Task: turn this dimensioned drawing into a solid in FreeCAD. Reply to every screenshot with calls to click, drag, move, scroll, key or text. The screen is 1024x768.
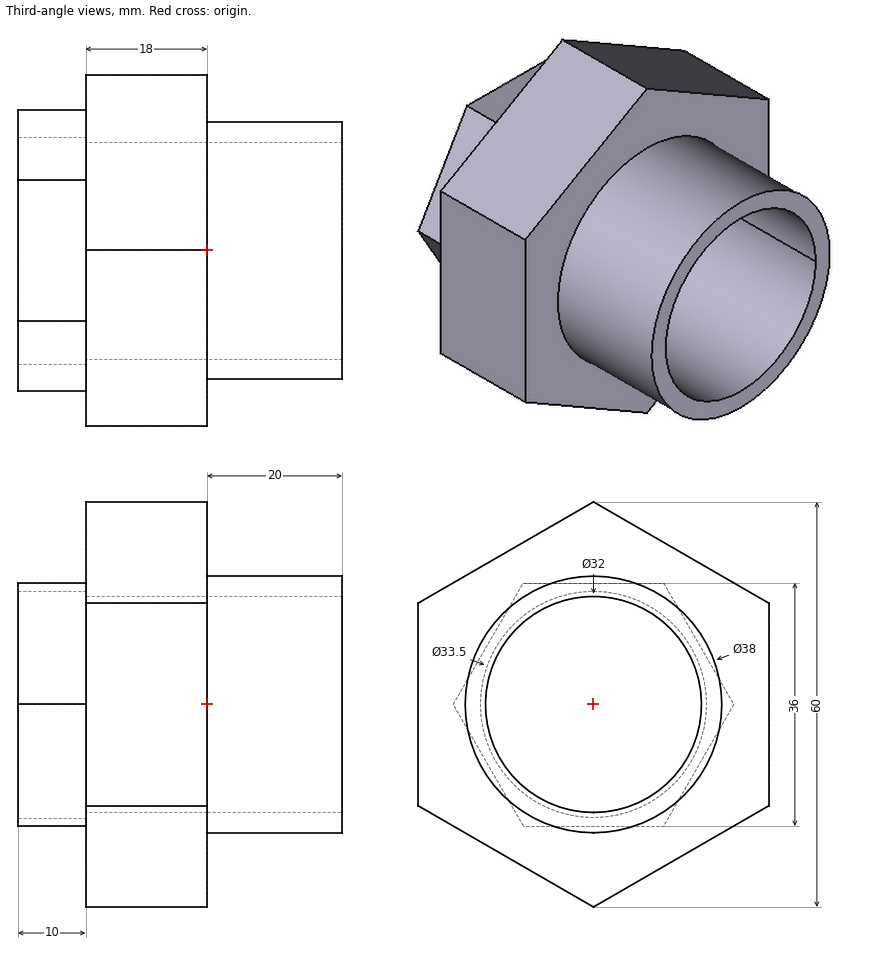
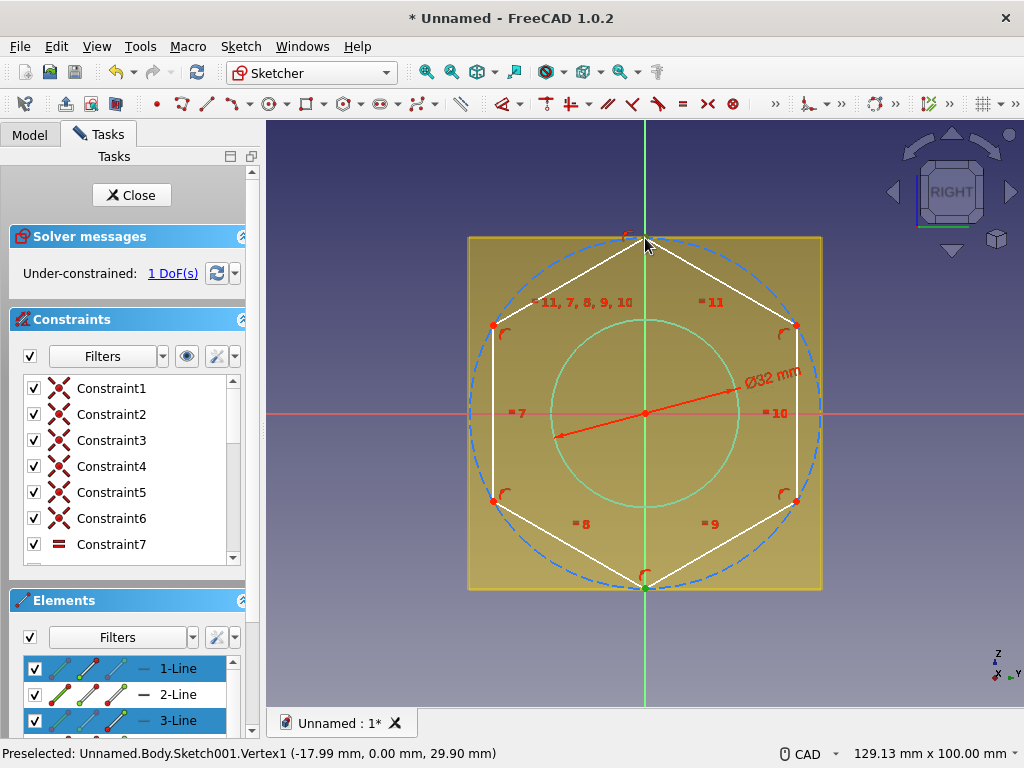
key(i)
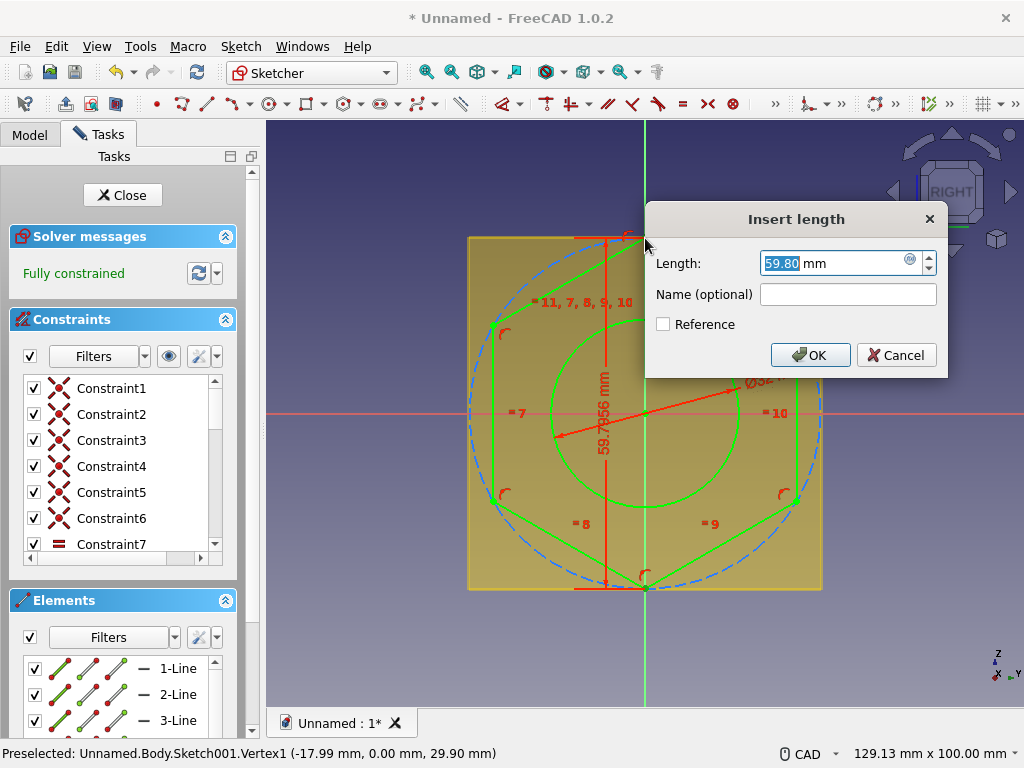
text(60)
key(Return)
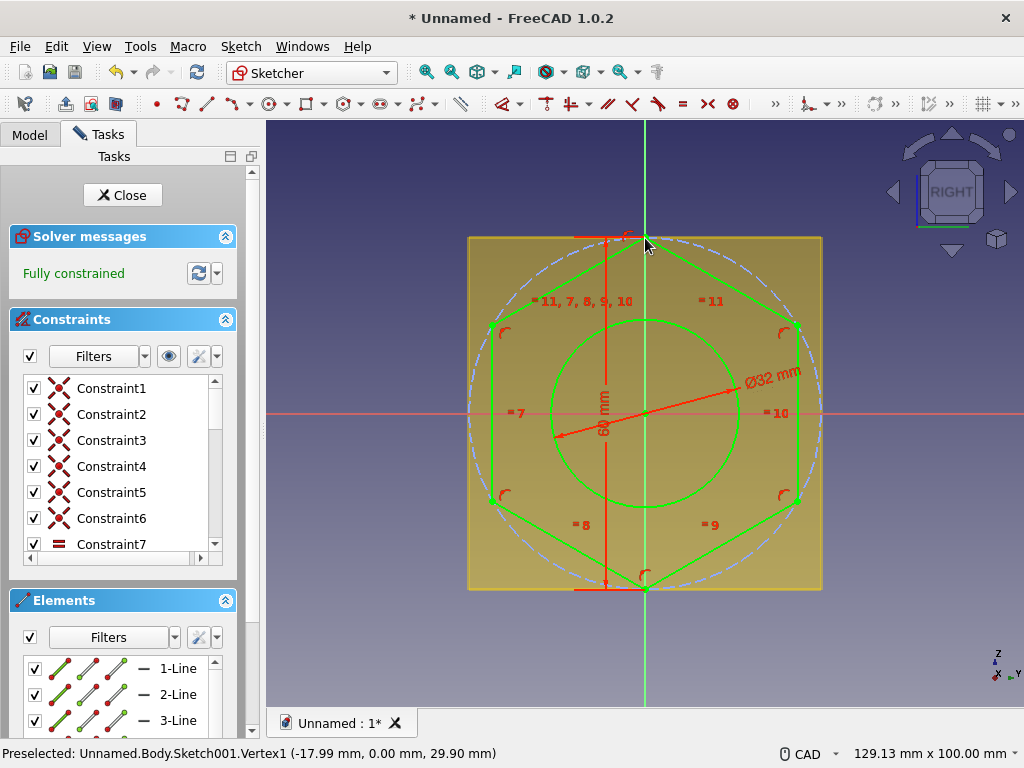
click(123, 195)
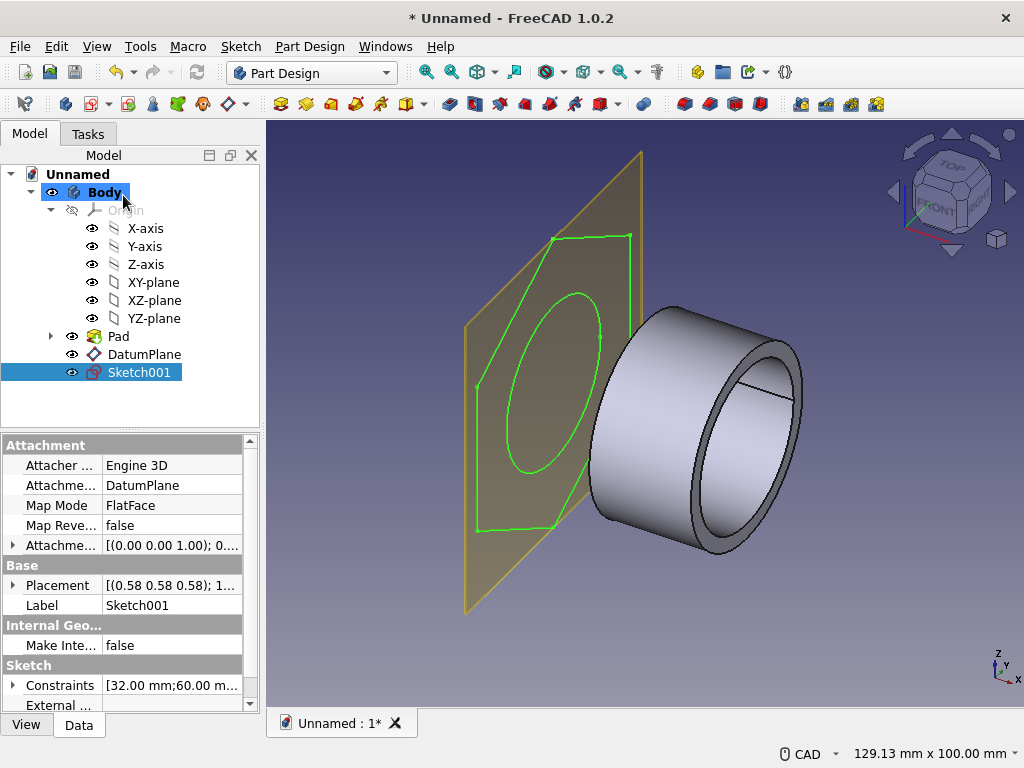
click(281, 104)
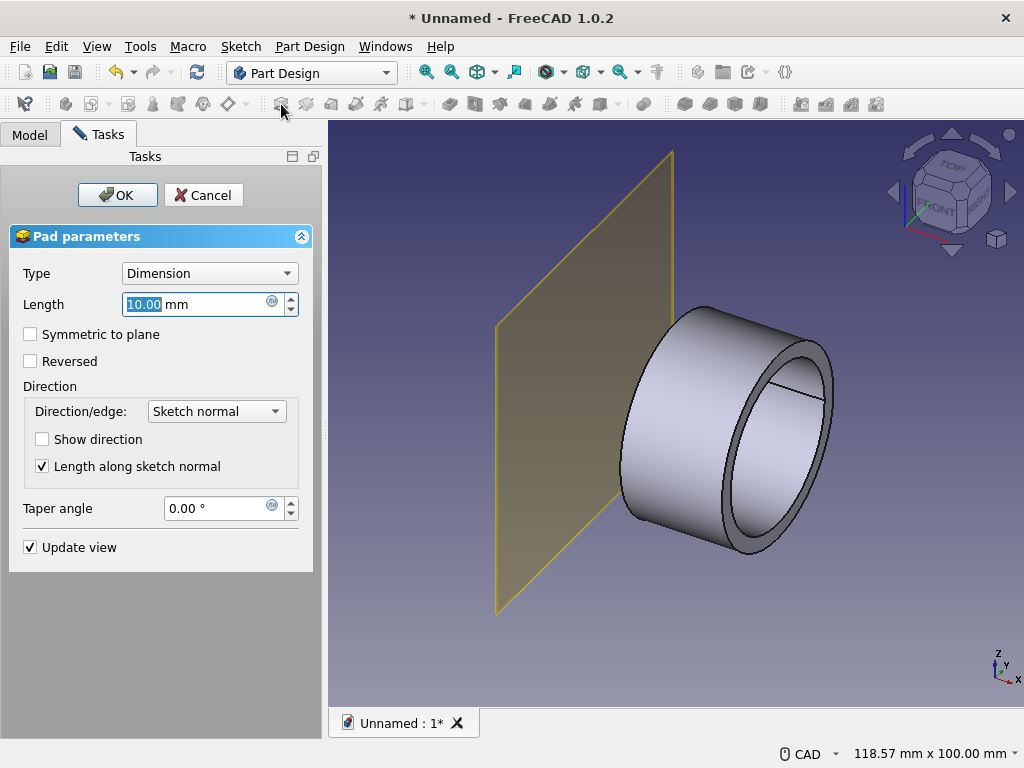
text(18)
key(Tab)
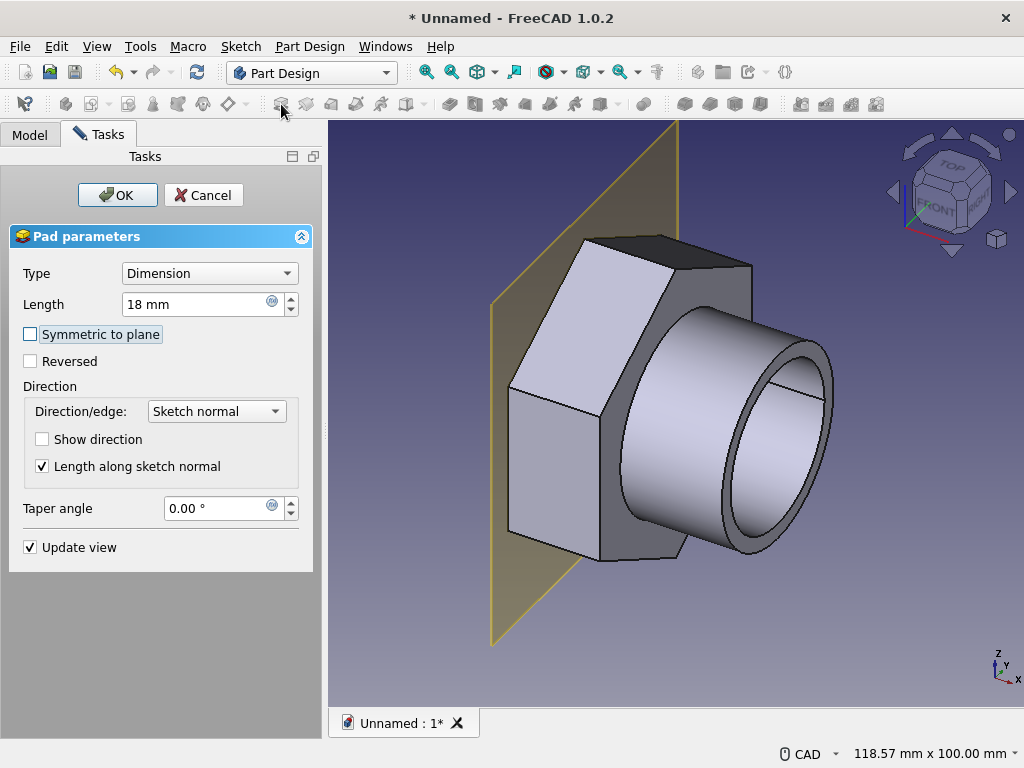
click(118, 195)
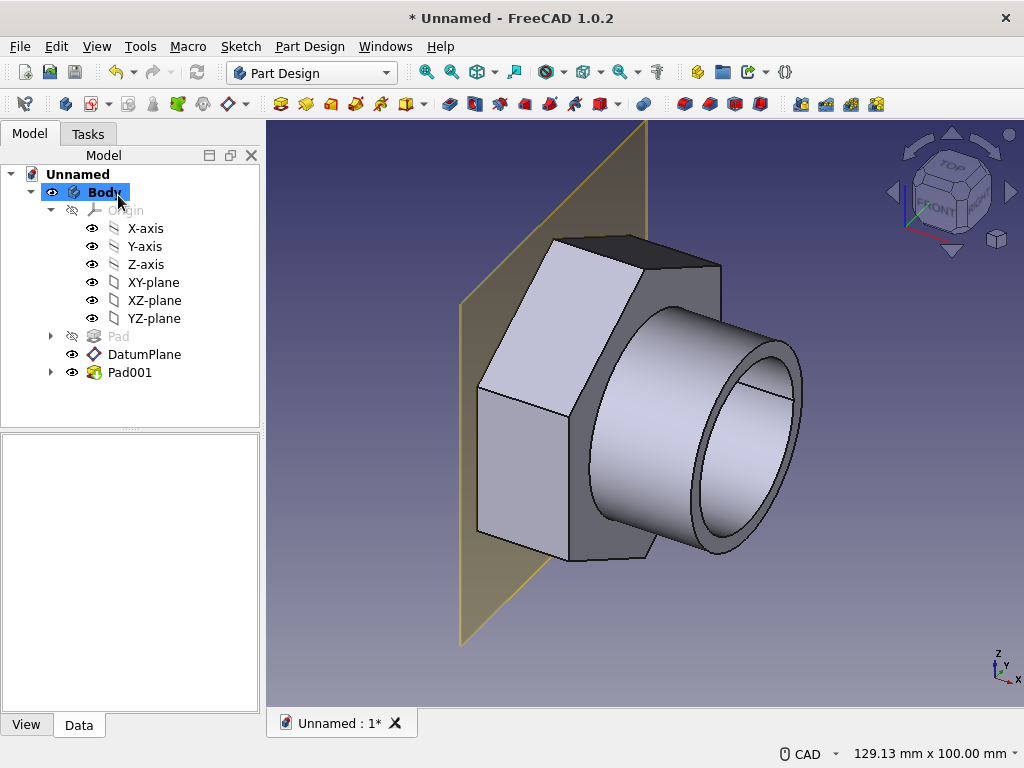
click(117, 354)
key(space)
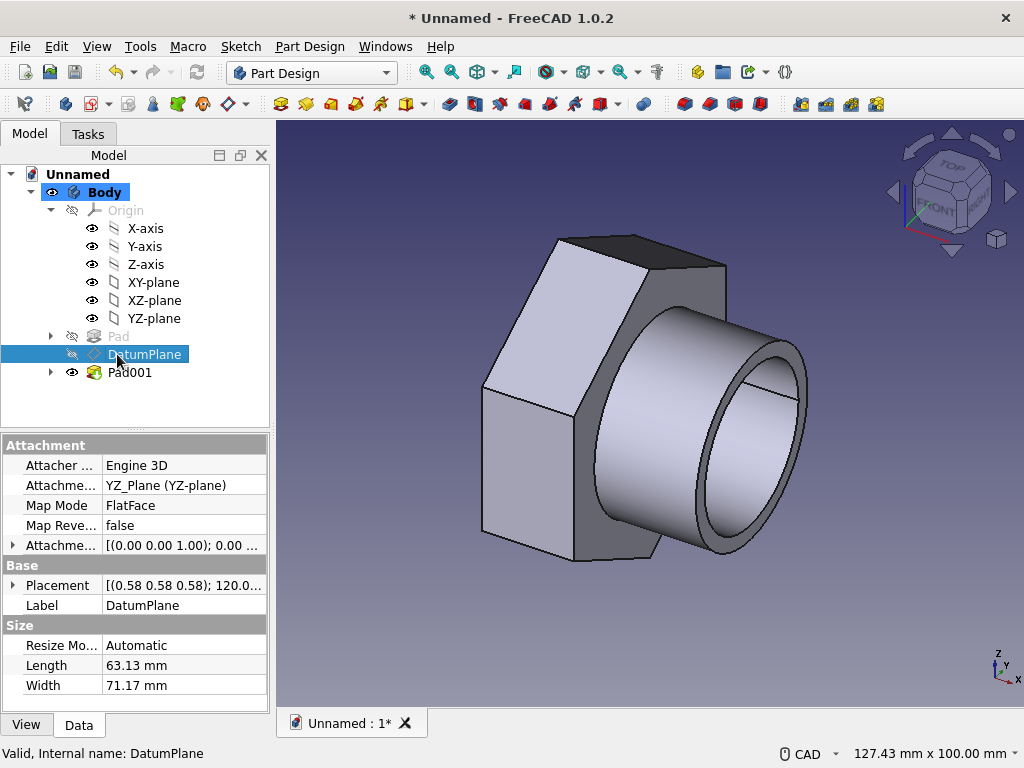
key(6)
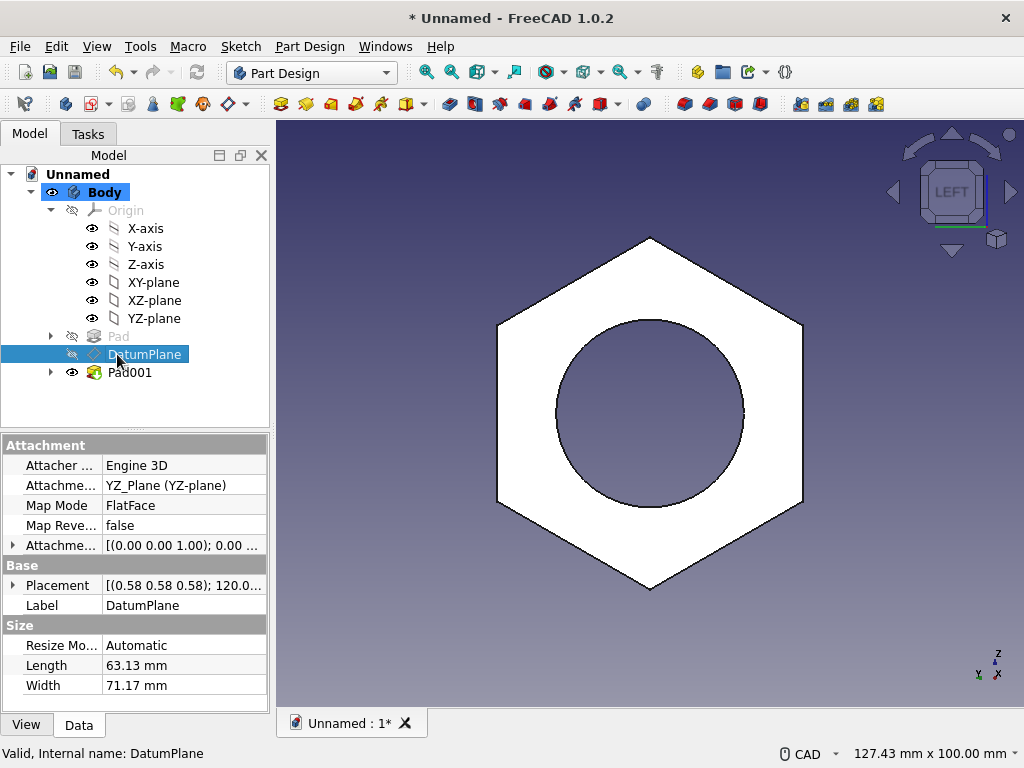
click(563, 513)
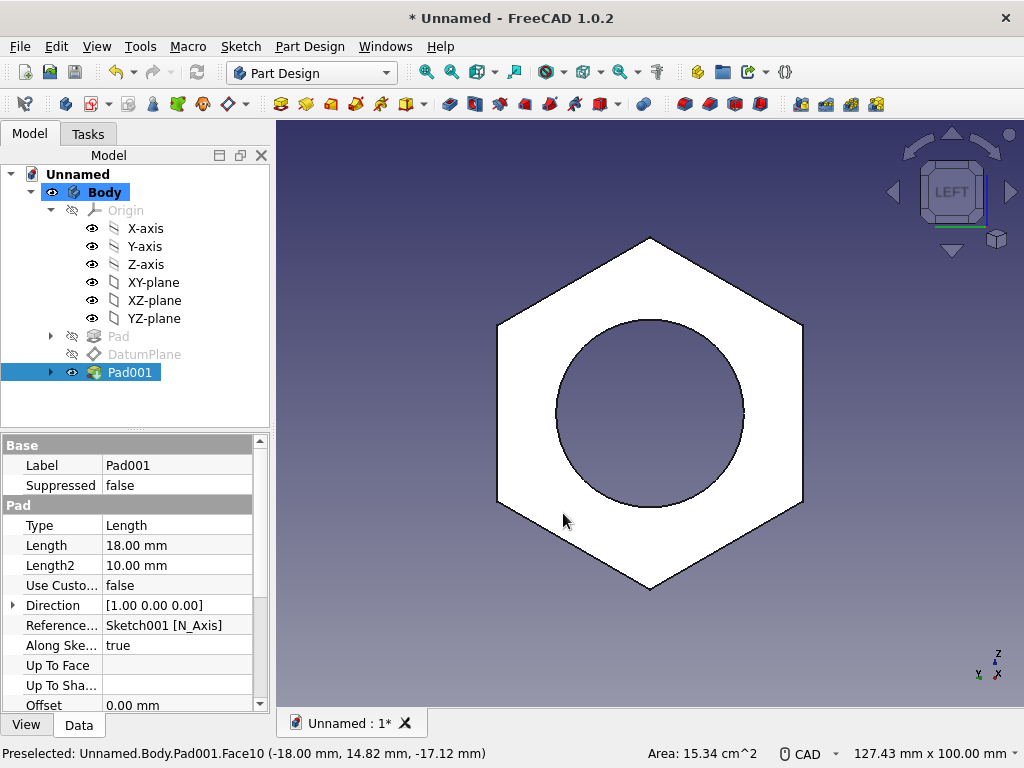
click(90, 104)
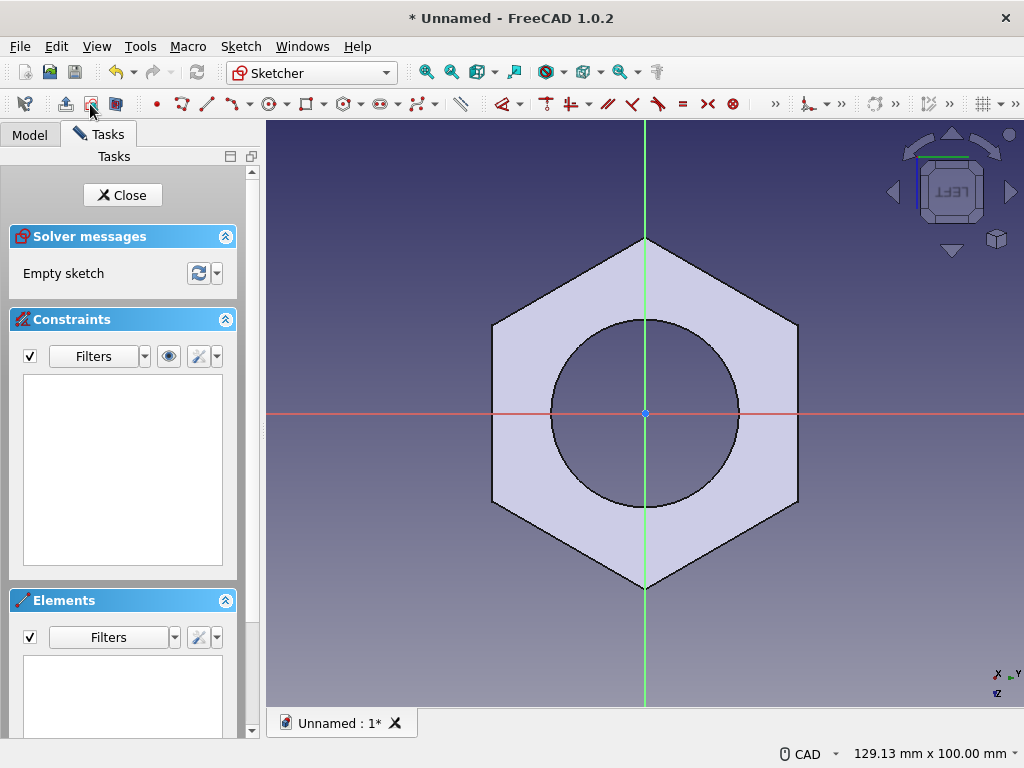
scroll(784, 413, up, 2)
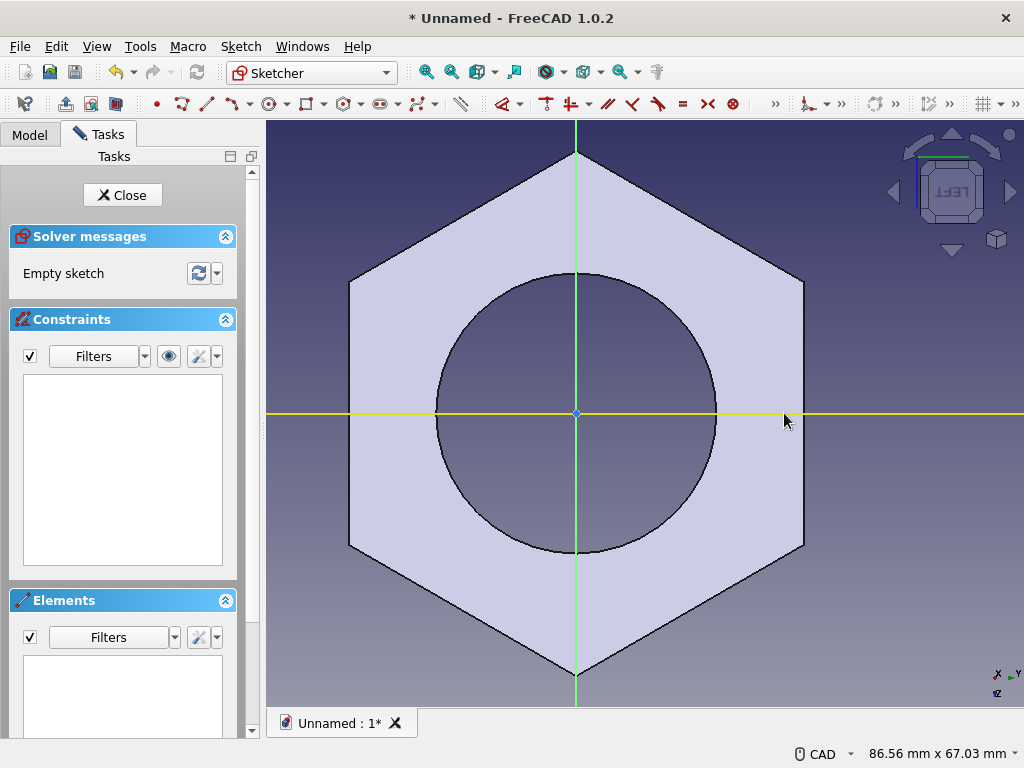
key(g)
key(p)
key(6)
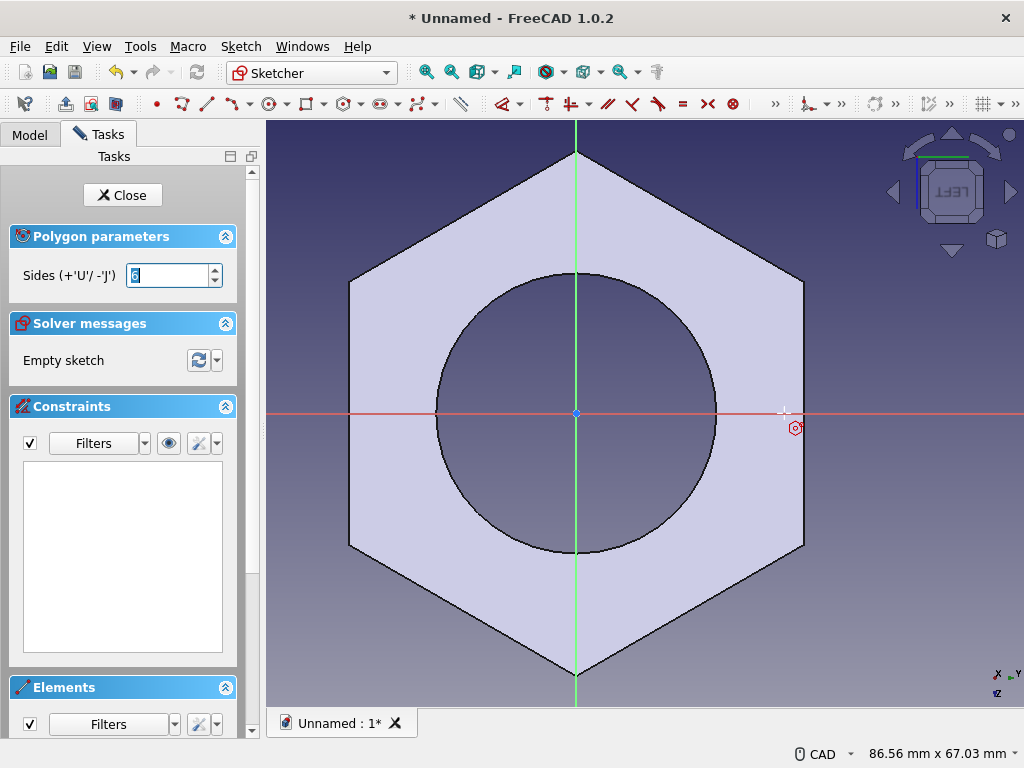
click(576, 414)